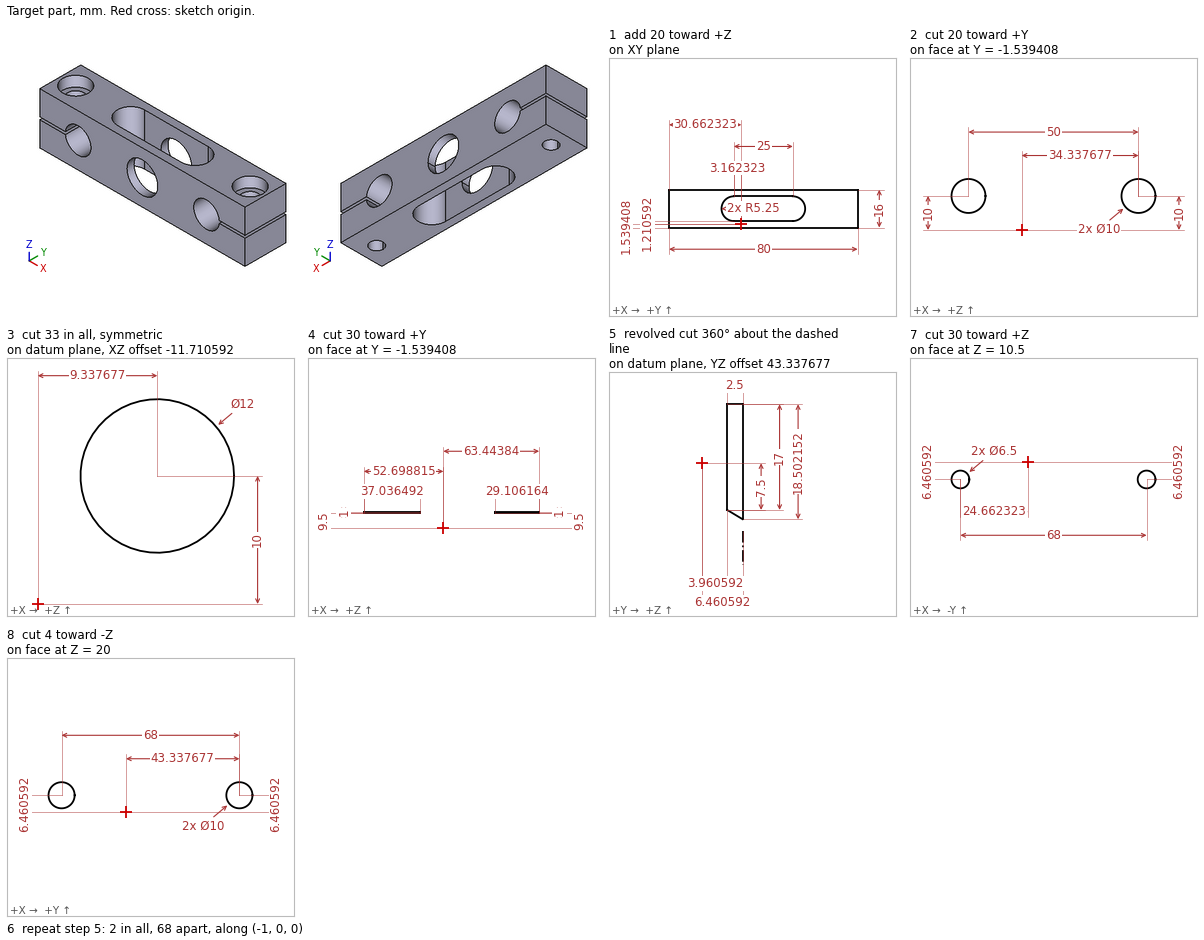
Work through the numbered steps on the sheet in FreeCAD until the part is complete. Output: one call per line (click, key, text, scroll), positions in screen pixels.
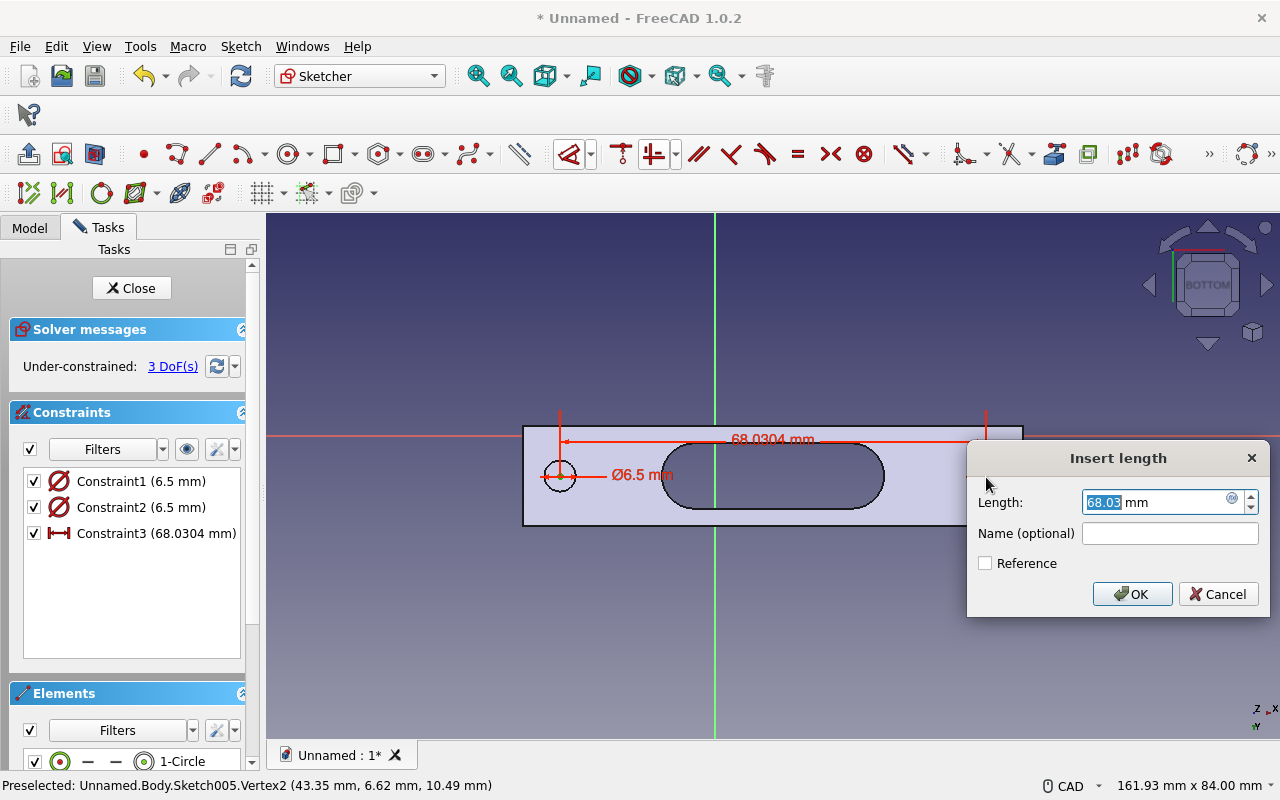
text(68)
key(Return)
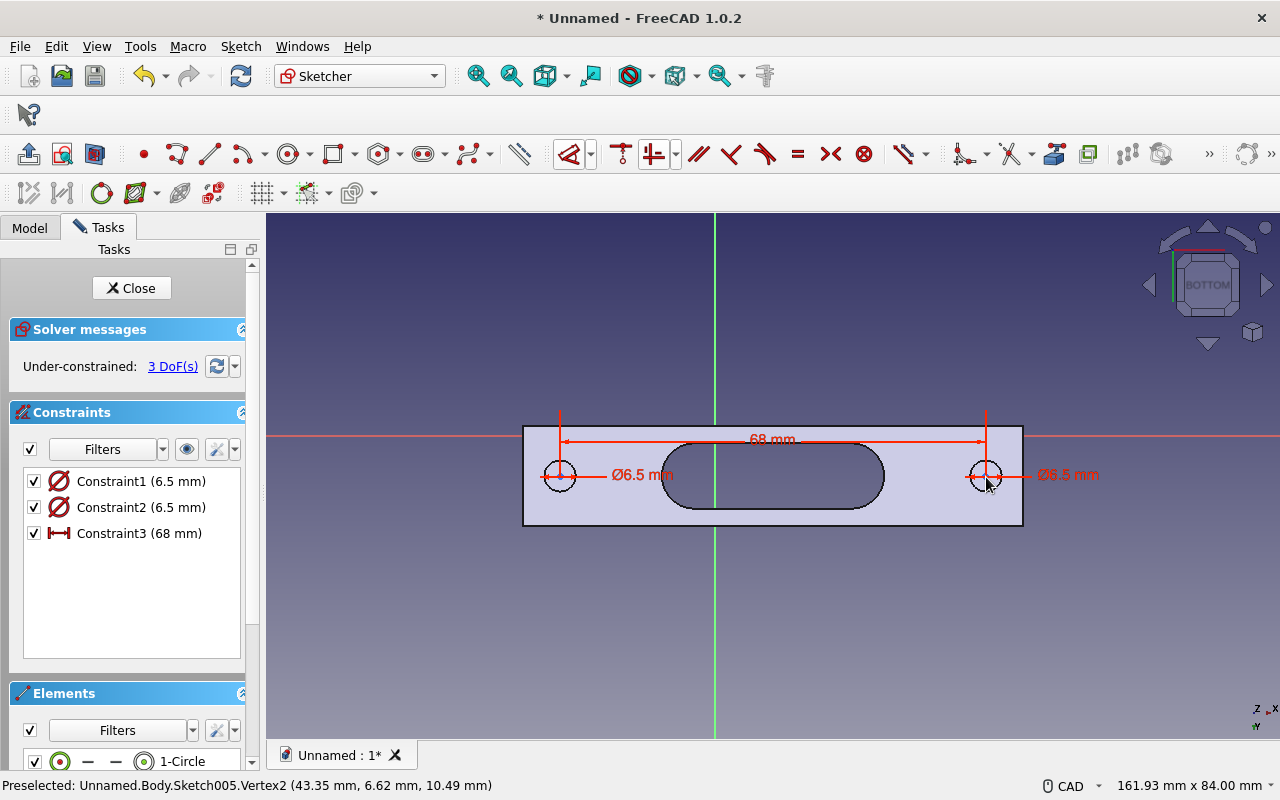
click(560, 477)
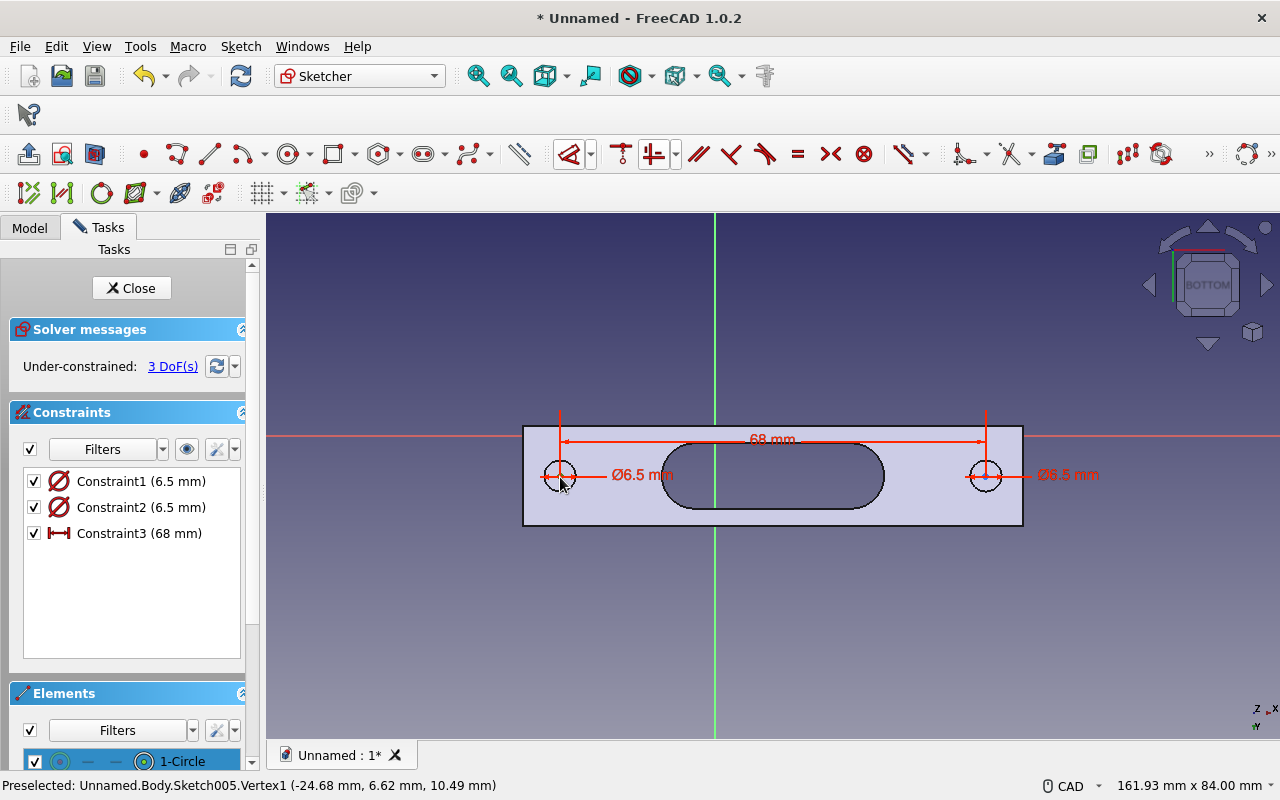
key(i)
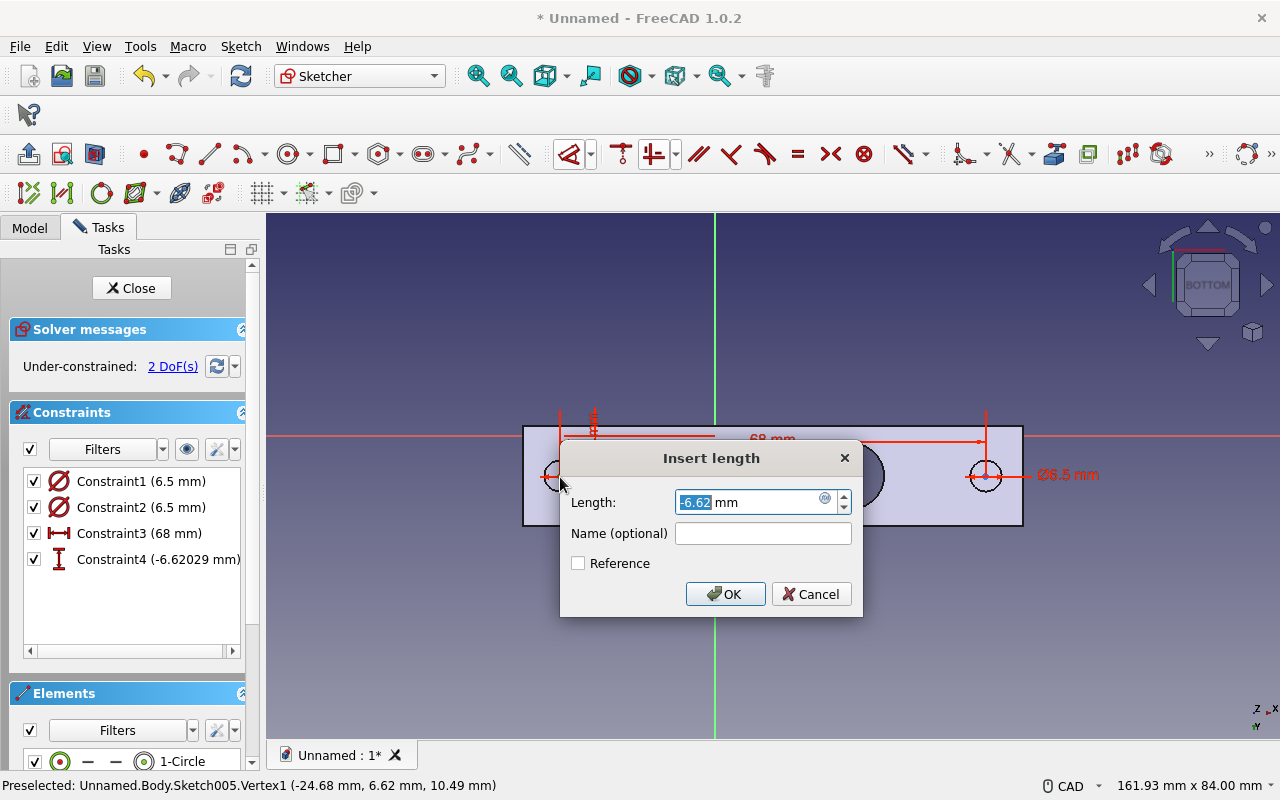
text(-6.460592)
key(Return)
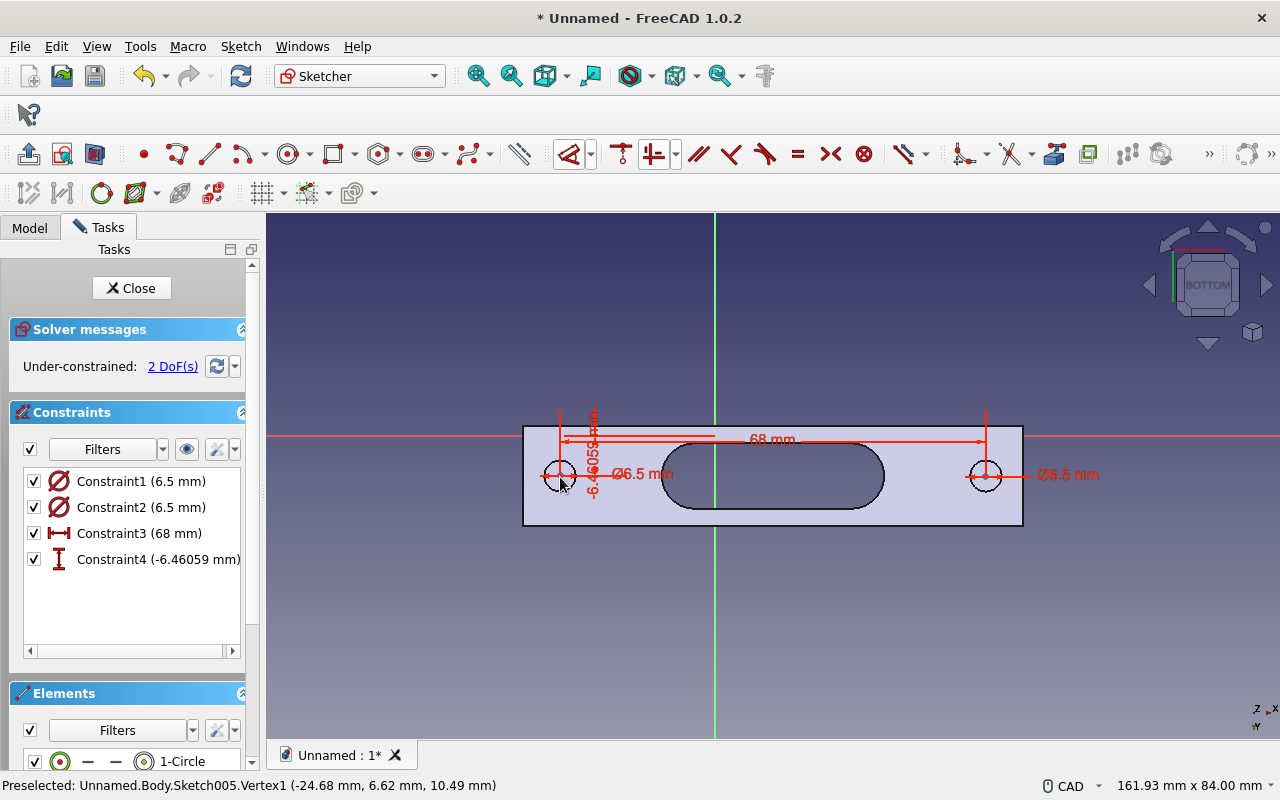
click(986, 477)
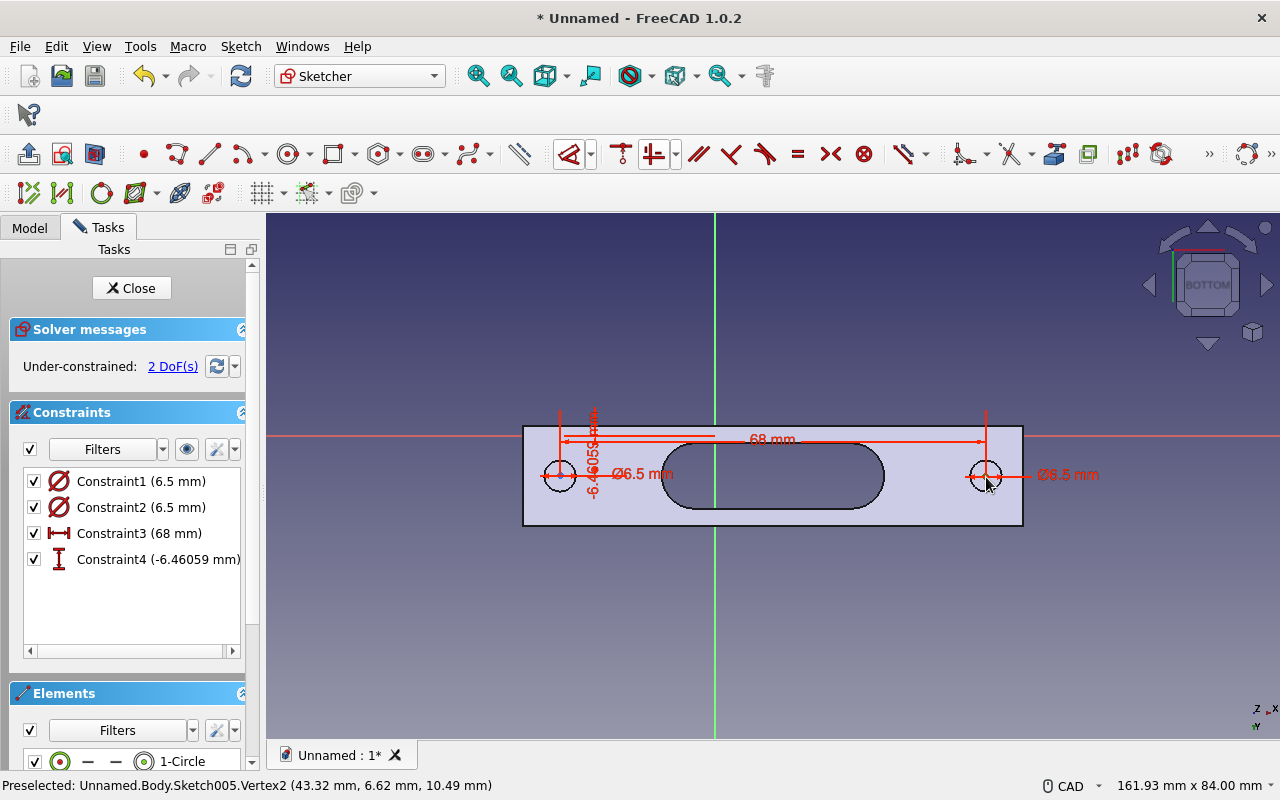
key(i)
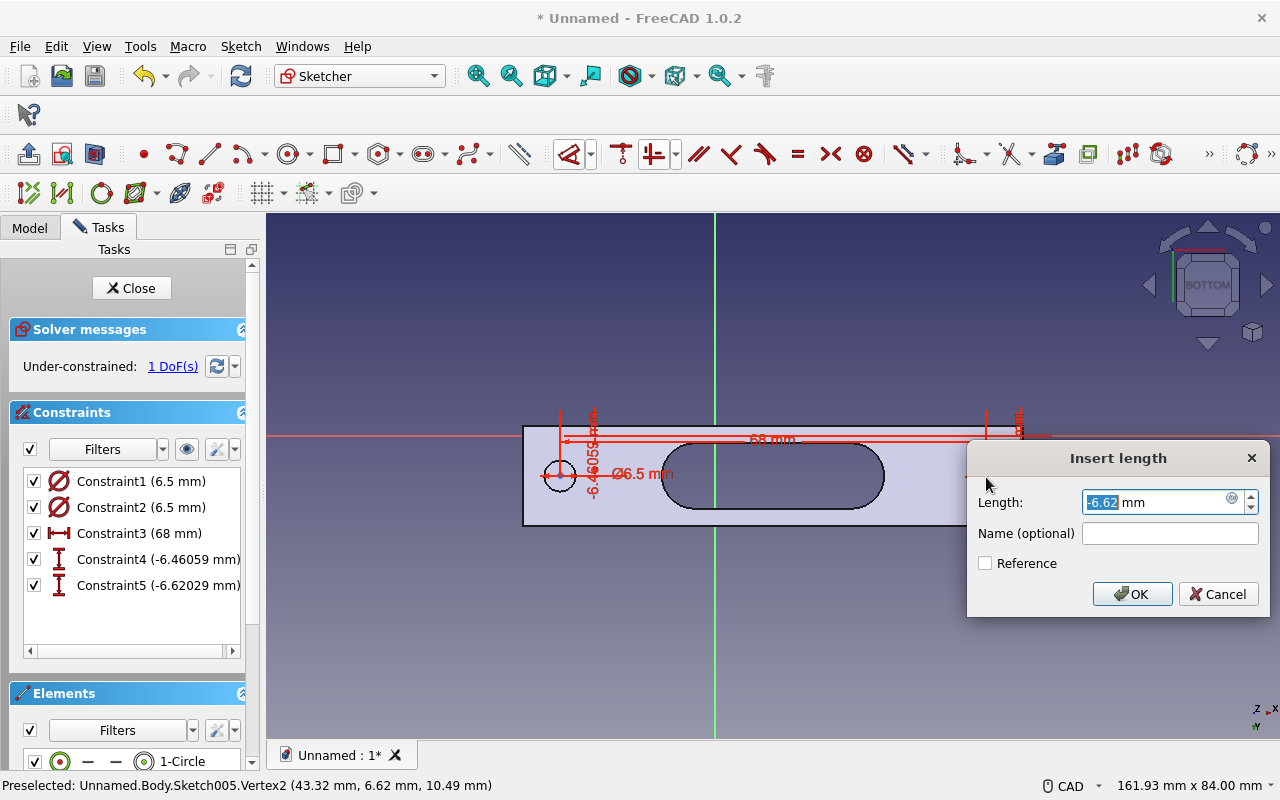
text(-6.460592)
key(Return)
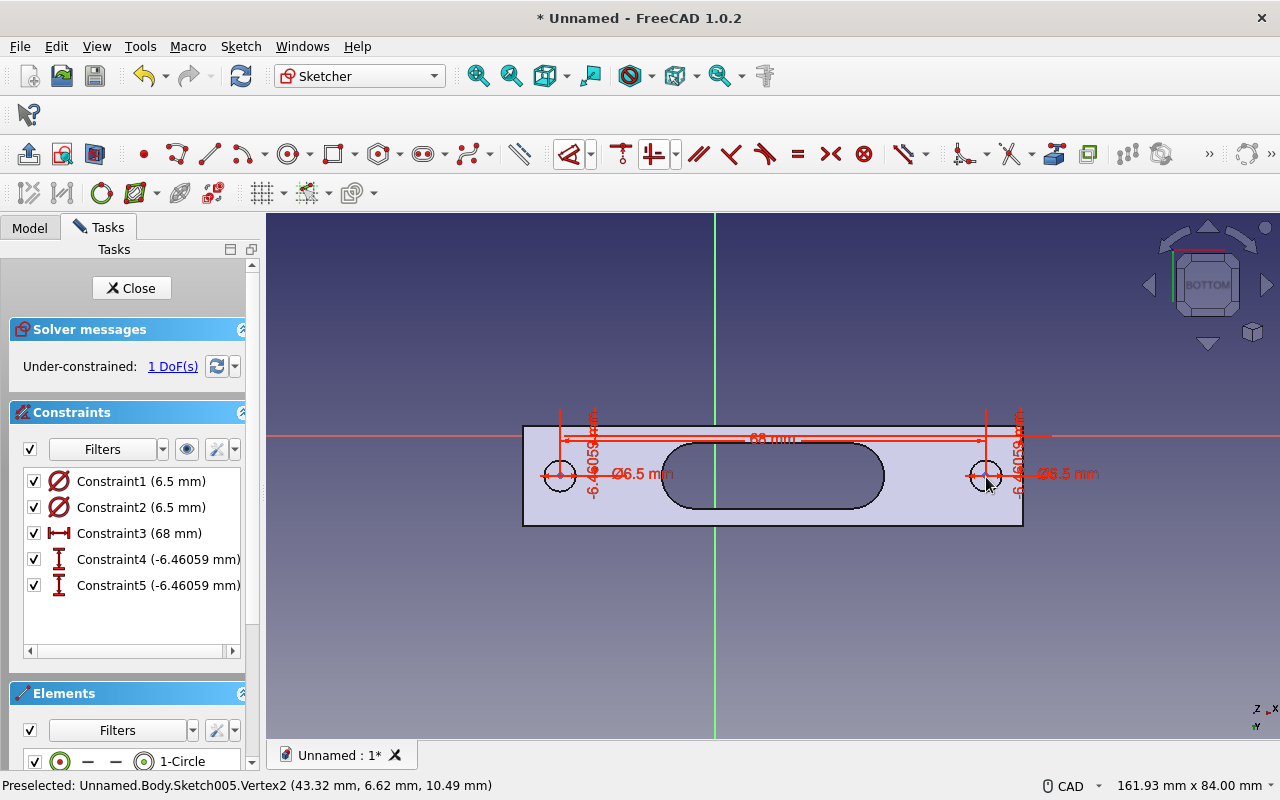
click(560, 476)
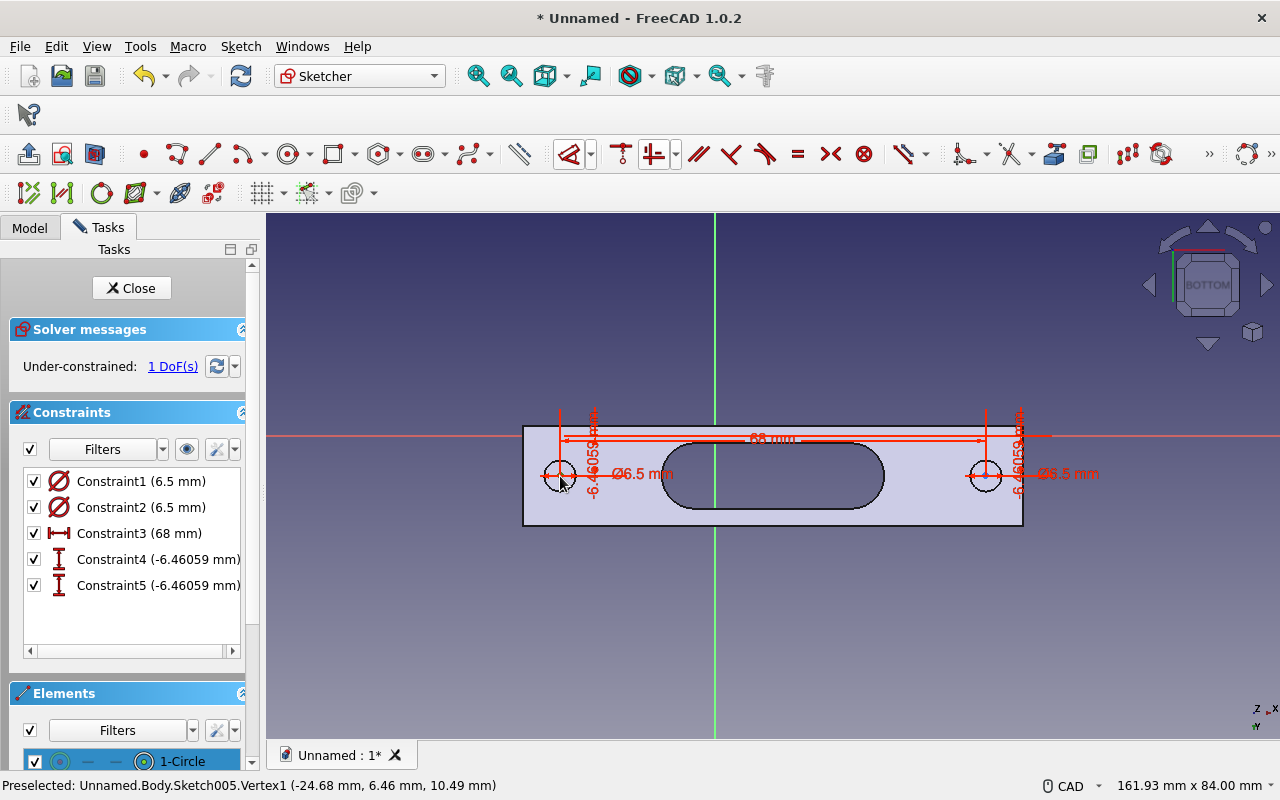
key(l)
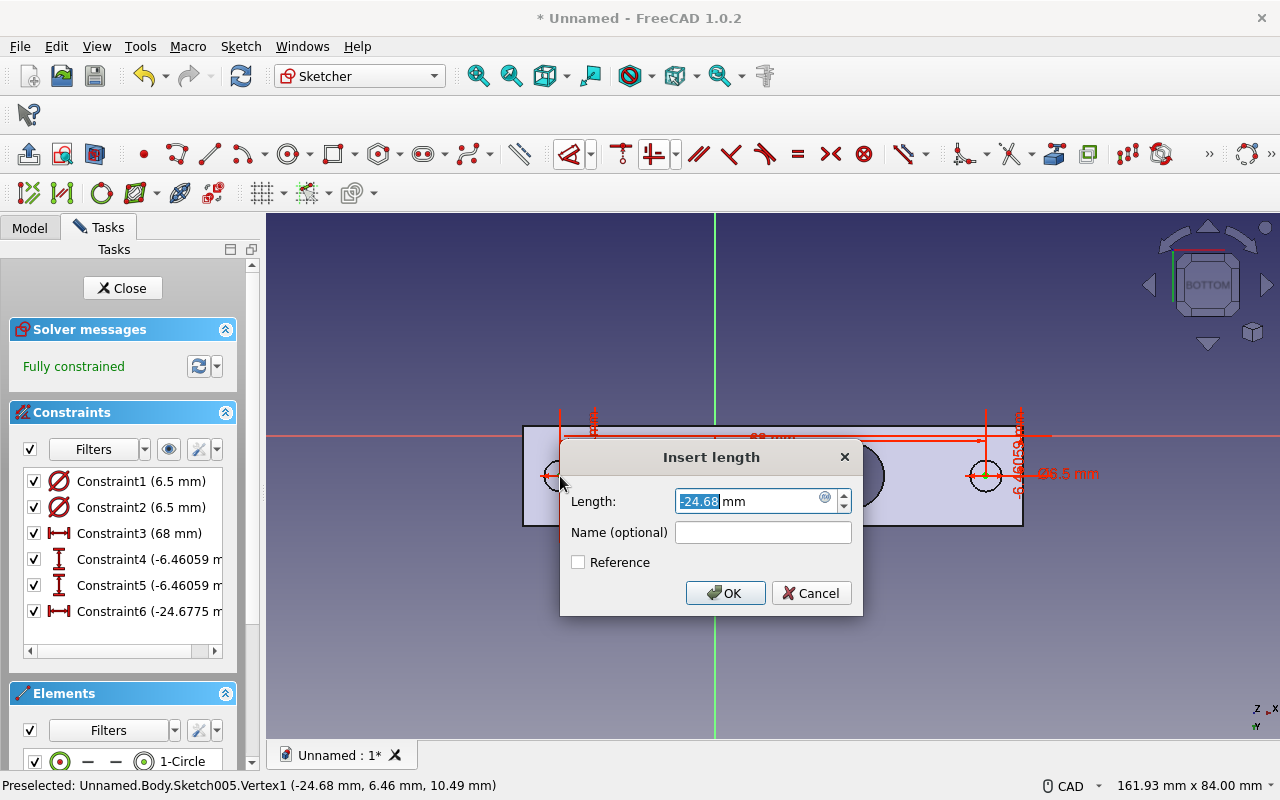
text(-24.662323)
key(Return)